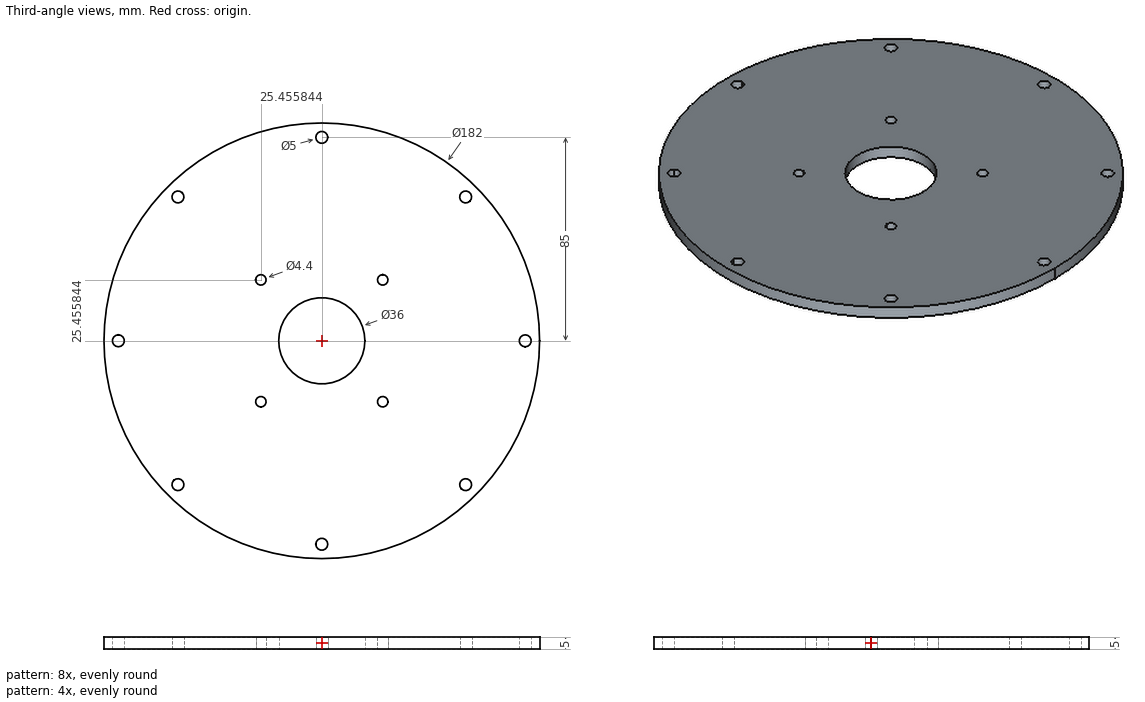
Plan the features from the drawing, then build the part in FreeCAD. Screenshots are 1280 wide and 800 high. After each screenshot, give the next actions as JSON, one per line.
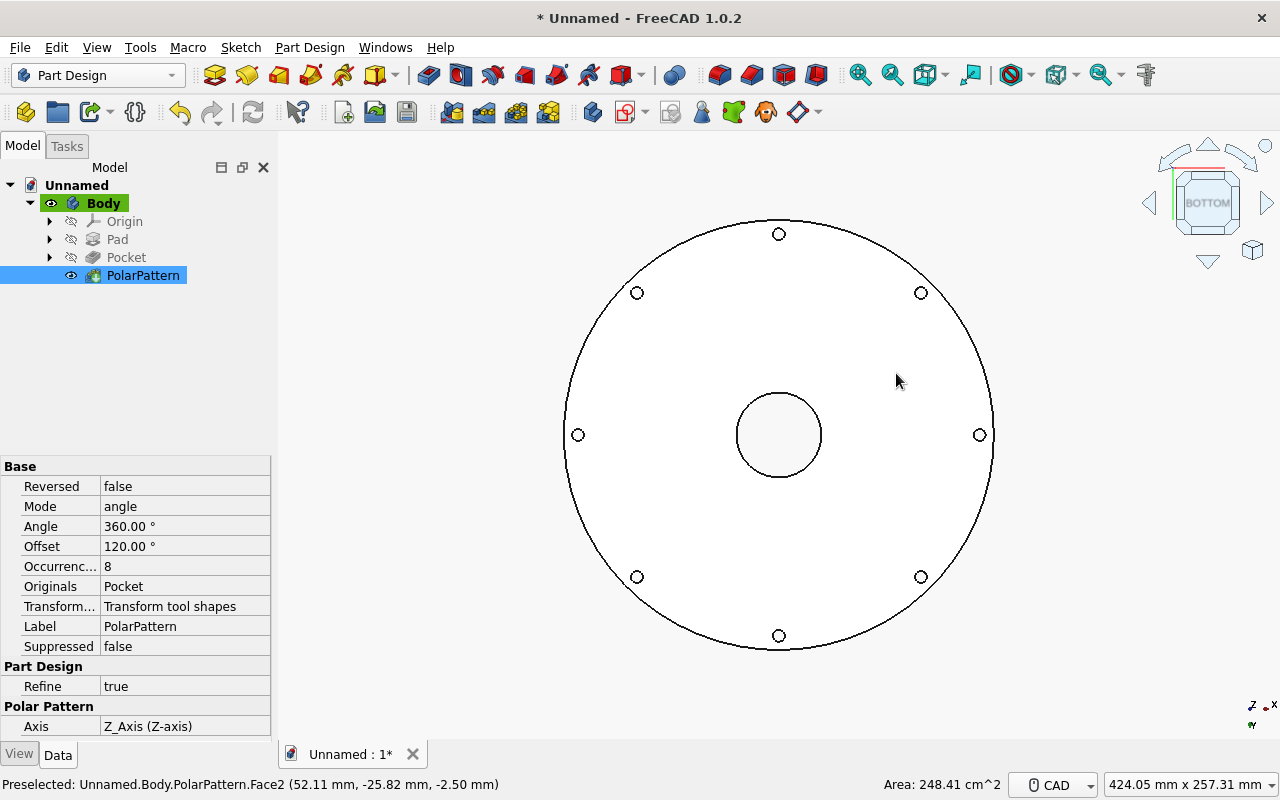
{"action": "left_click", "coordinate": [626, 112]}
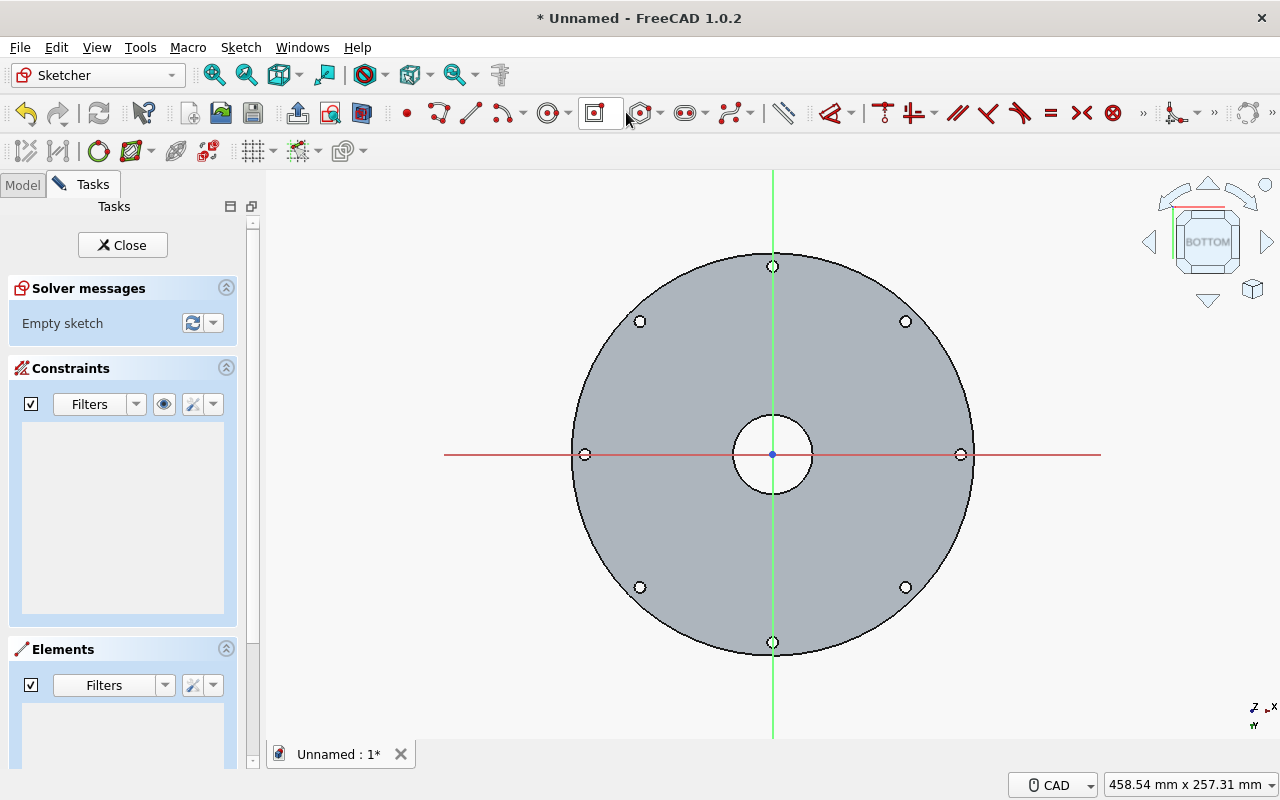
{"action": "scroll", "coordinate": [717, 514], "scroll_direction": "up", "scroll_amount": 15}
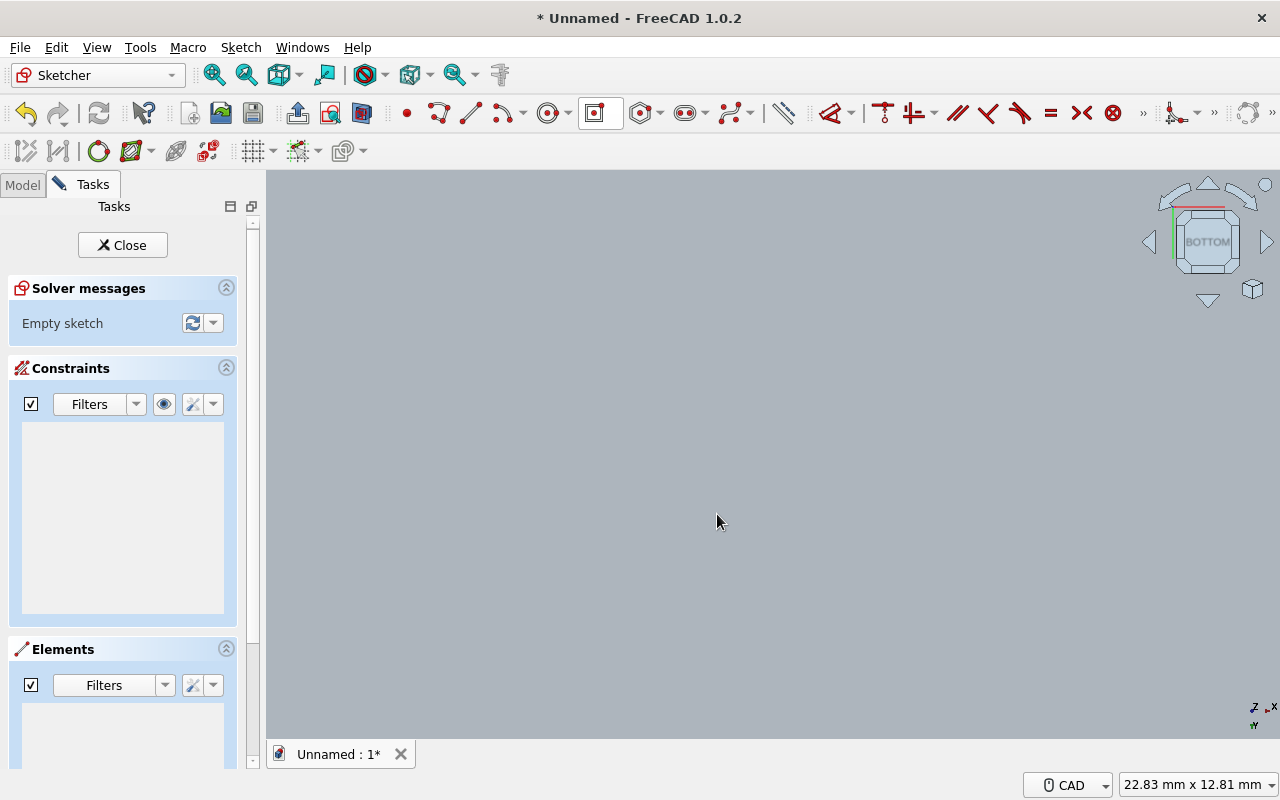
{"action": "scroll", "coordinate": [694, 418], "scroll_direction": "up", "scroll_amount": 3}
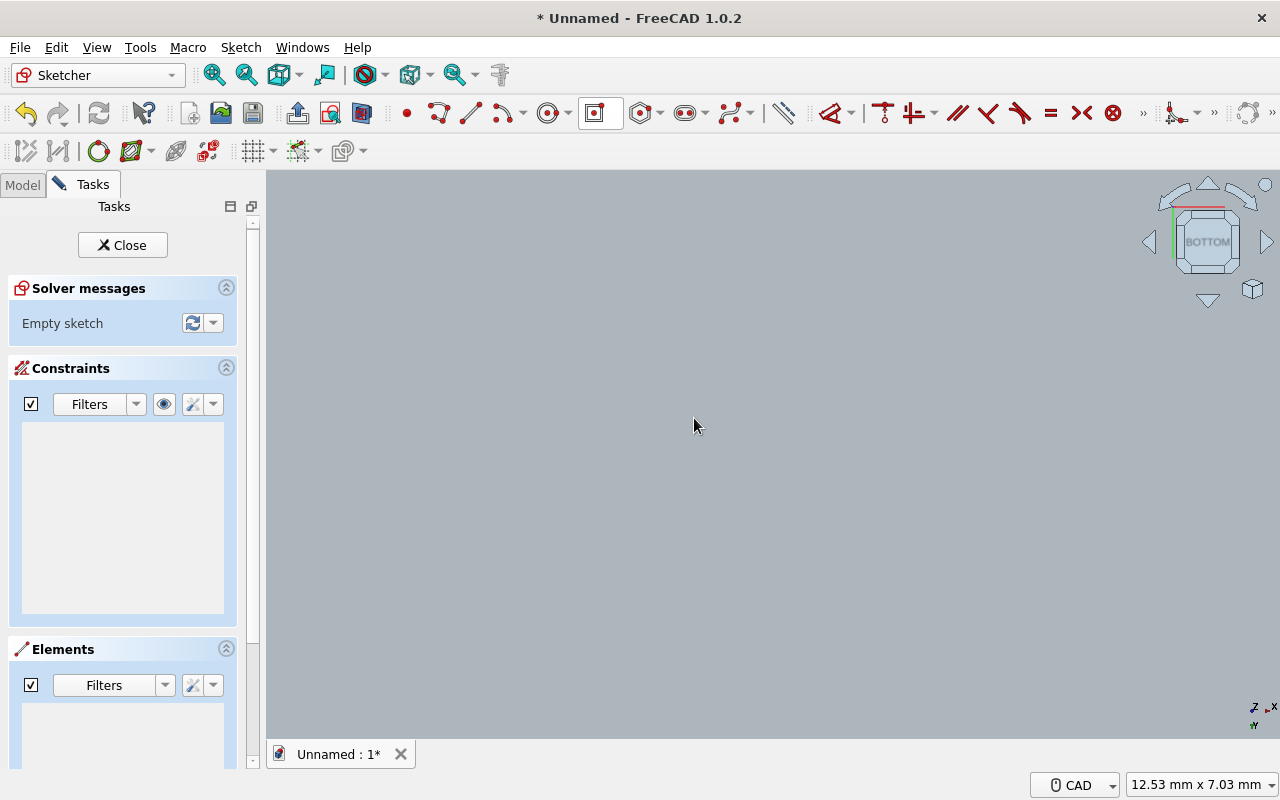
{"action": "left_click", "coordinate": [548, 114]}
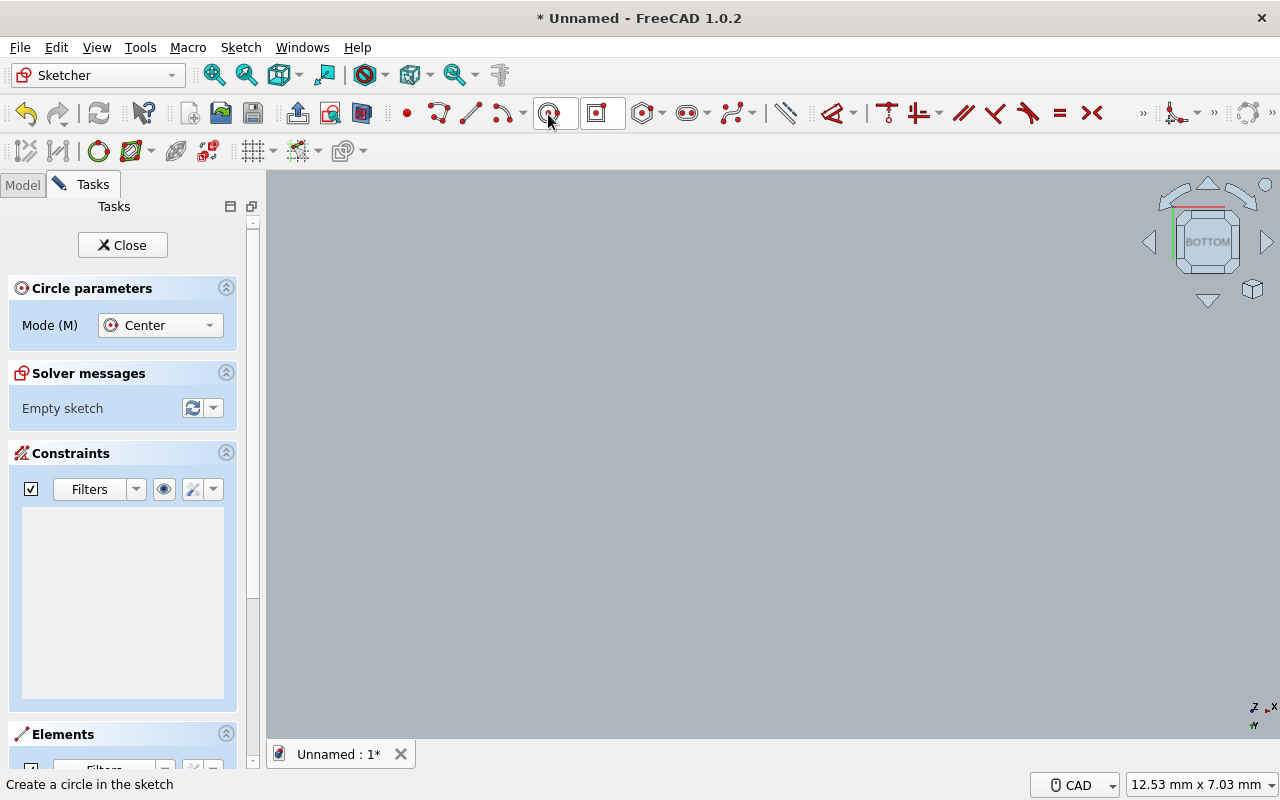
{"action": "left_click", "coordinate": [705, 454]}
{"action": "mouse_move", "coordinate": [830, 328]}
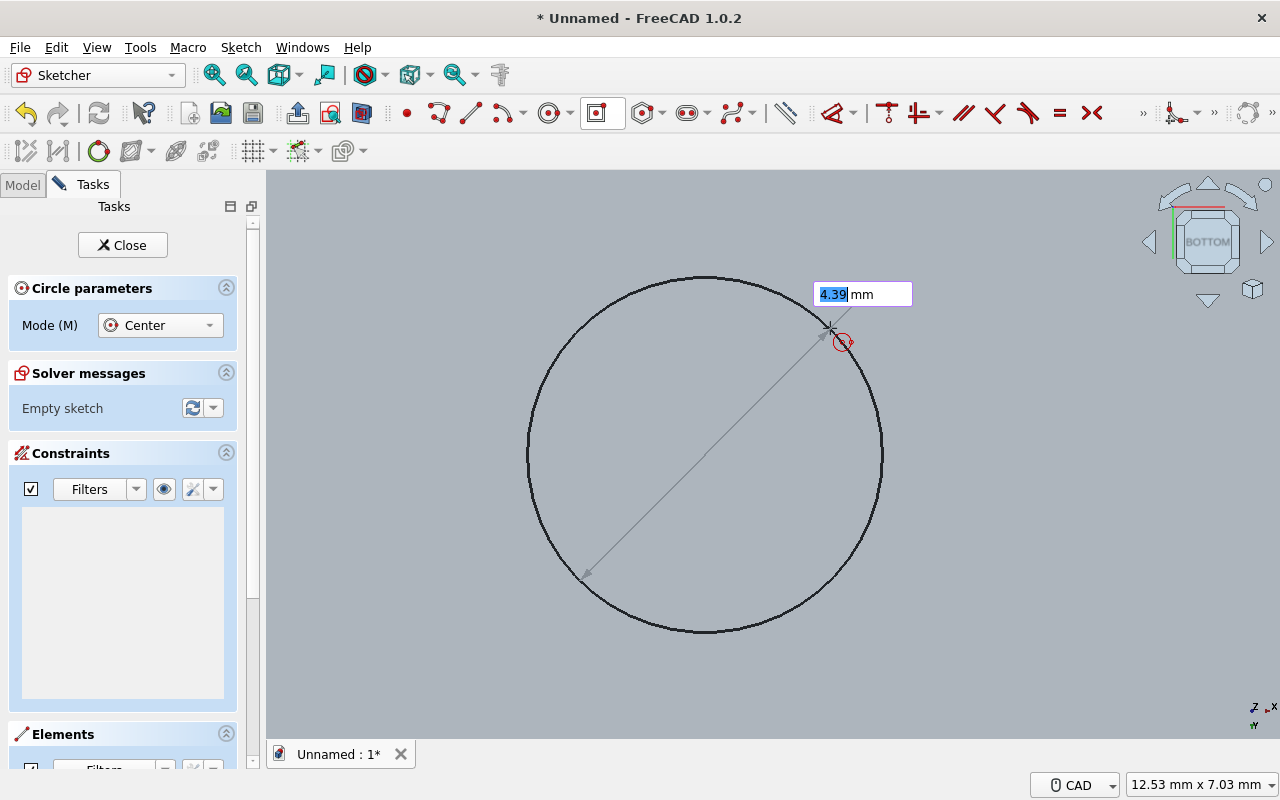
{"action": "type", "text": "4.4"}
{"action": "key", "text": "Return"}
{"action": "key", "text": "Escape"}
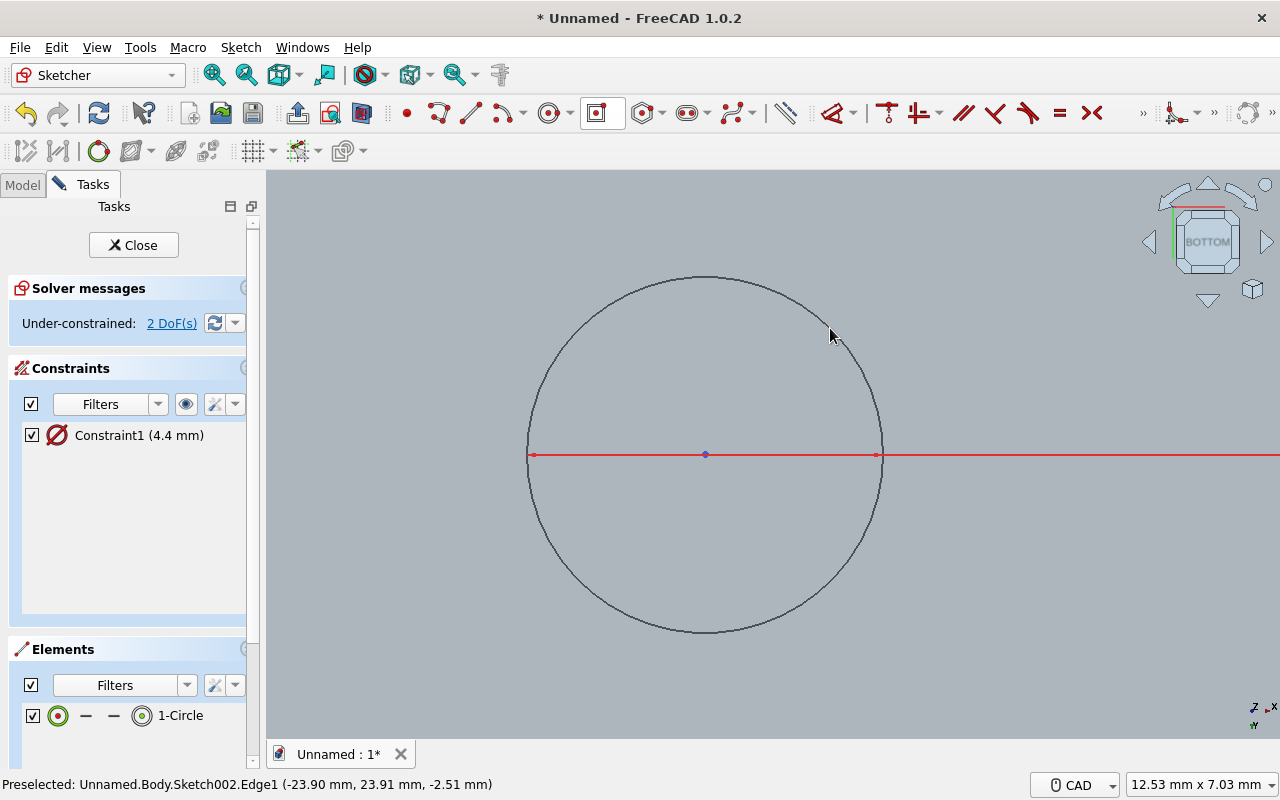
{"action": "left_click", "coordinate": [832, 114]}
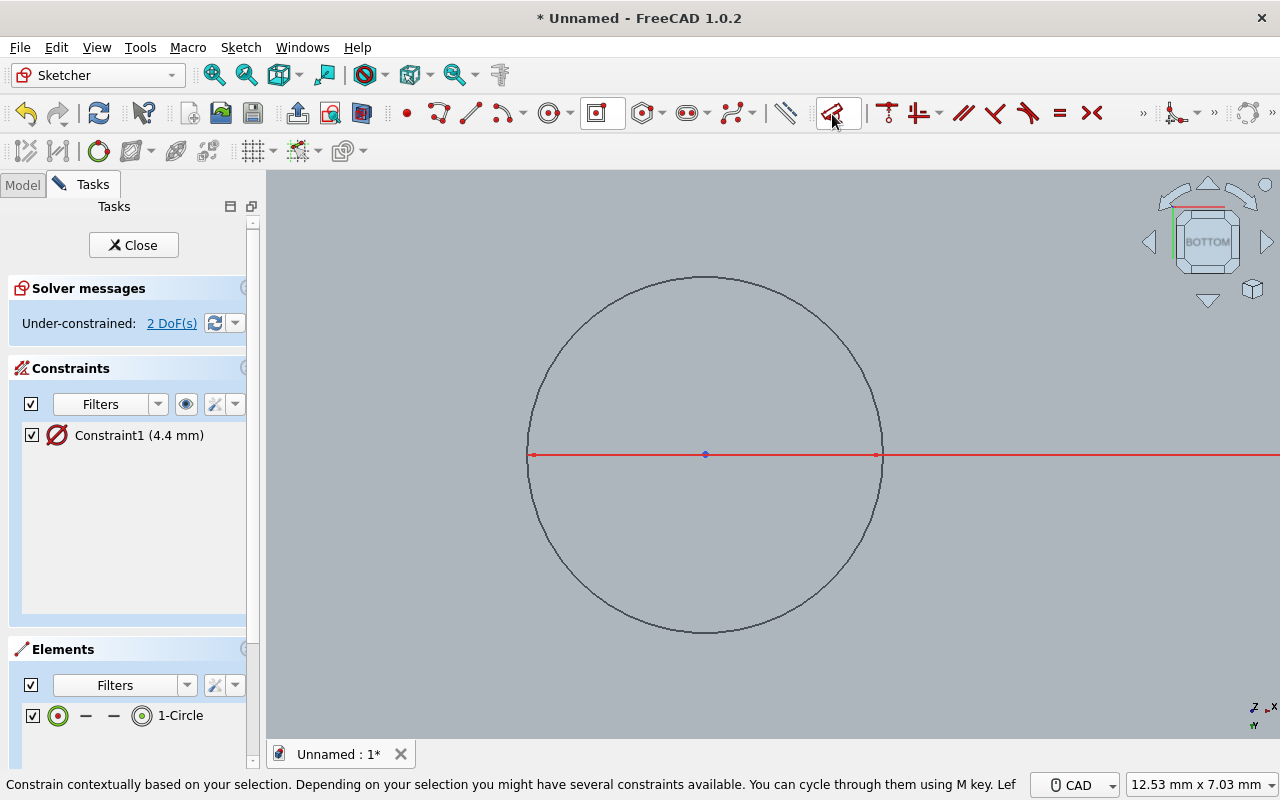
{"action": "left_click", "coordinate": [705, 455]}
{"action": "left_click", "coordinate": [910, 489]}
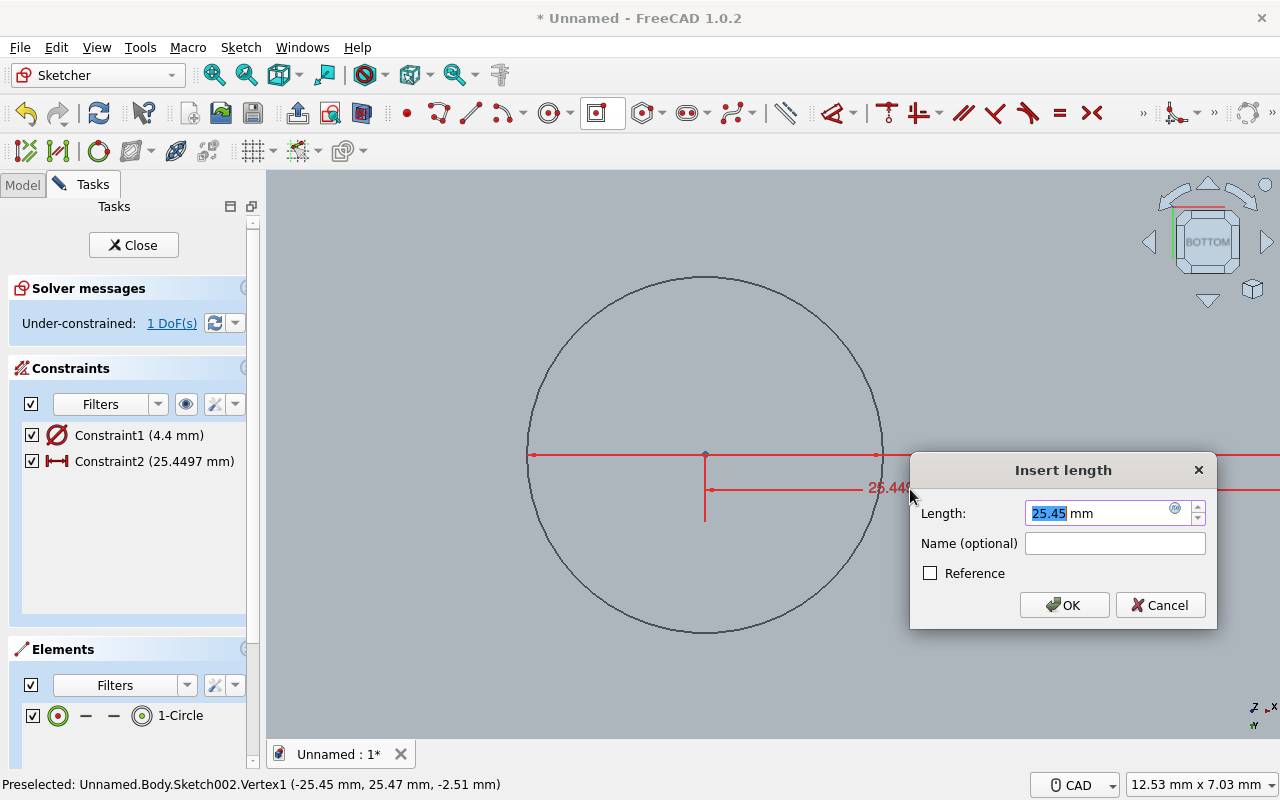
{"action": "type", "text": "25.455844"}
{"action": "key", "text": "Return"}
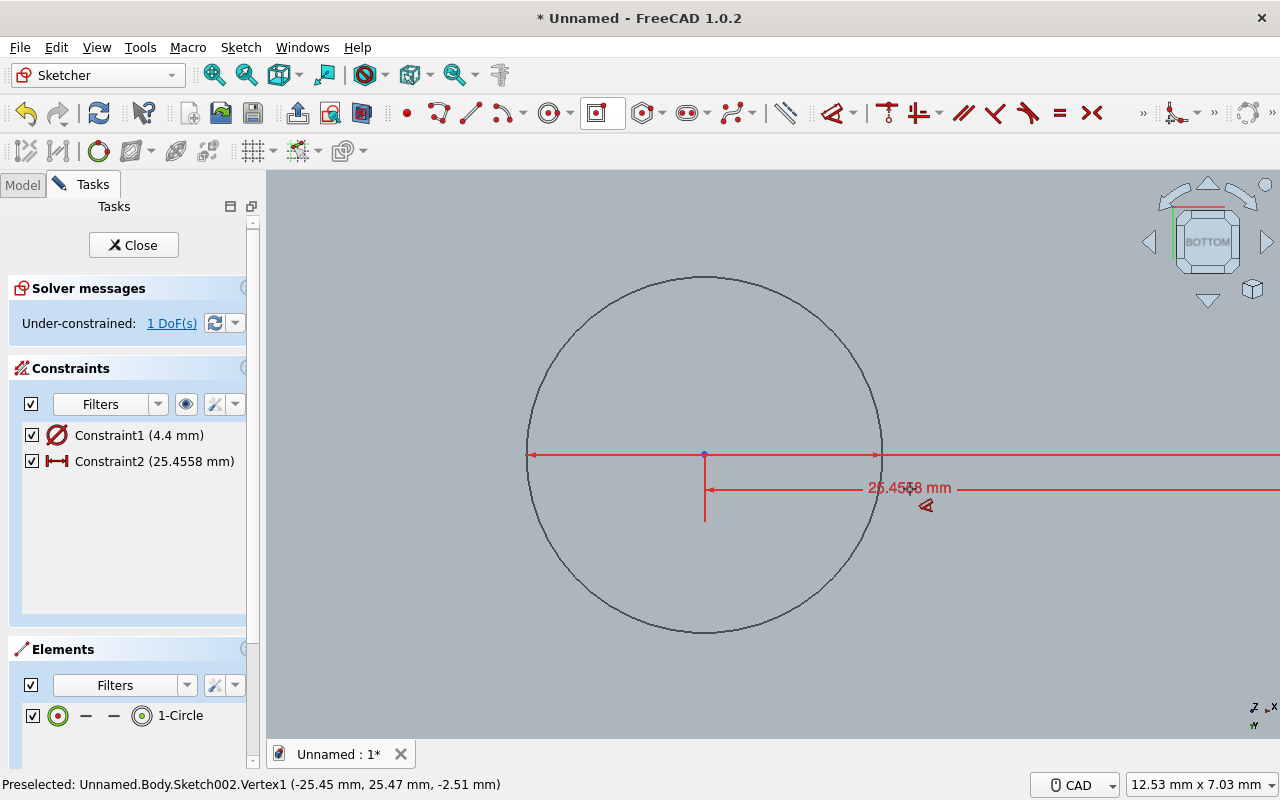
{"action": "left_click", "coordinate": [705, 455]}
{"action": "left_click", "coordinate": [671, 326]}